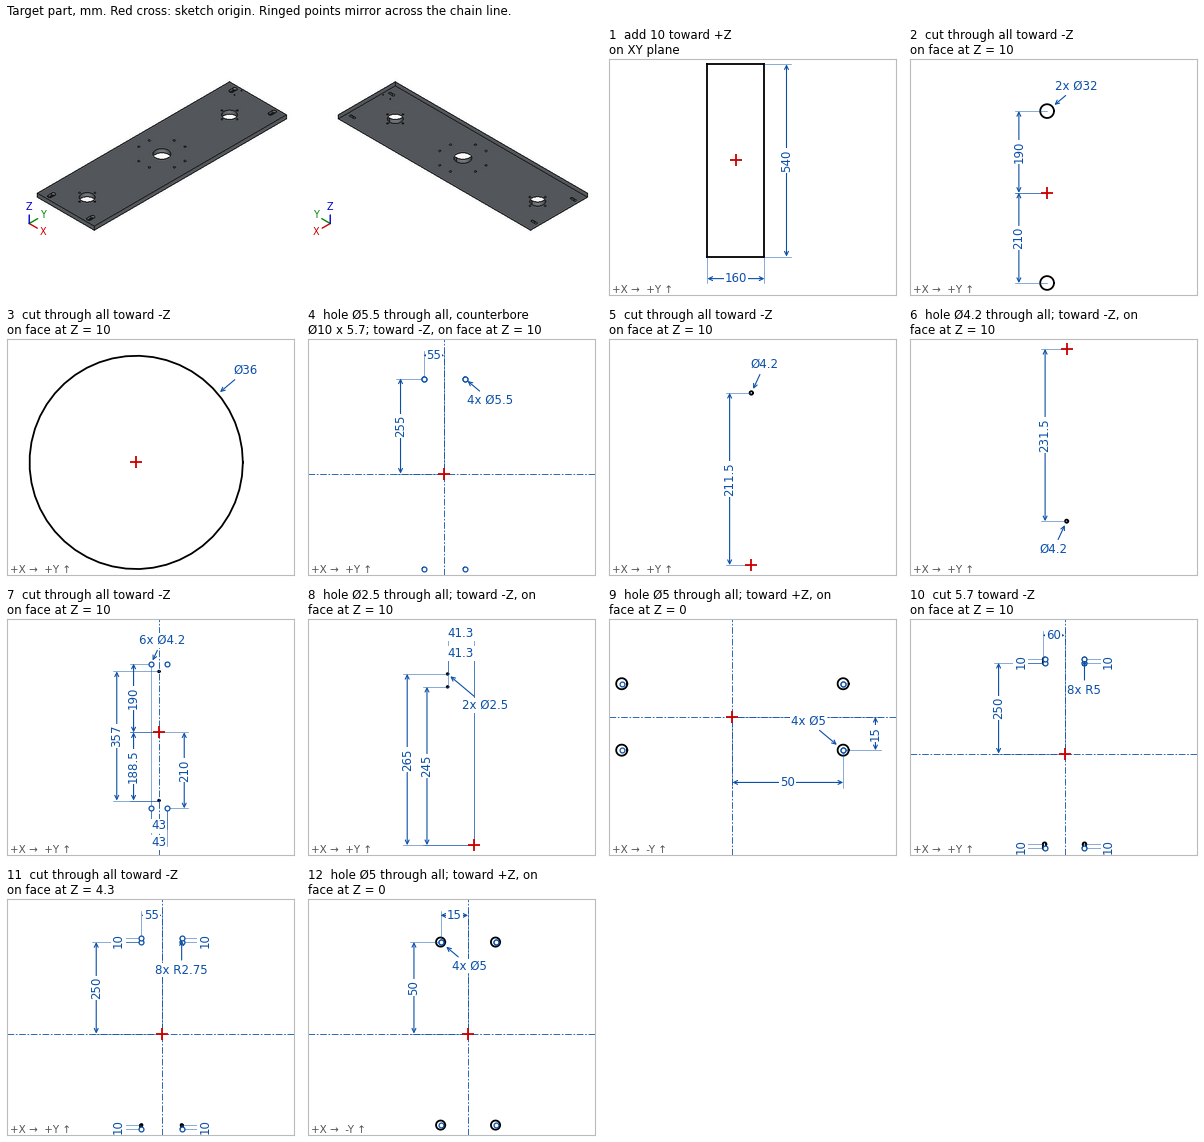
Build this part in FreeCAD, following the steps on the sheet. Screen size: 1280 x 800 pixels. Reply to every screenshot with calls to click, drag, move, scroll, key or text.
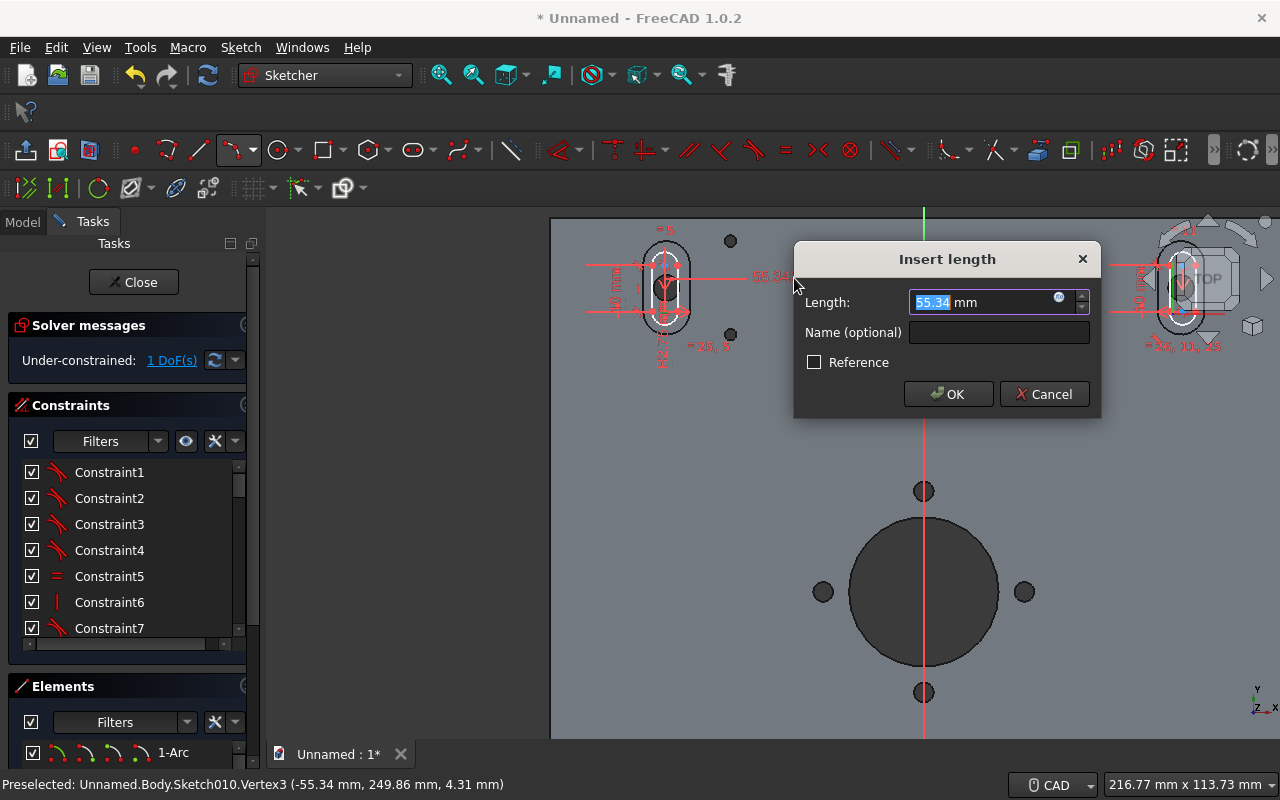
text(55)
key(Return)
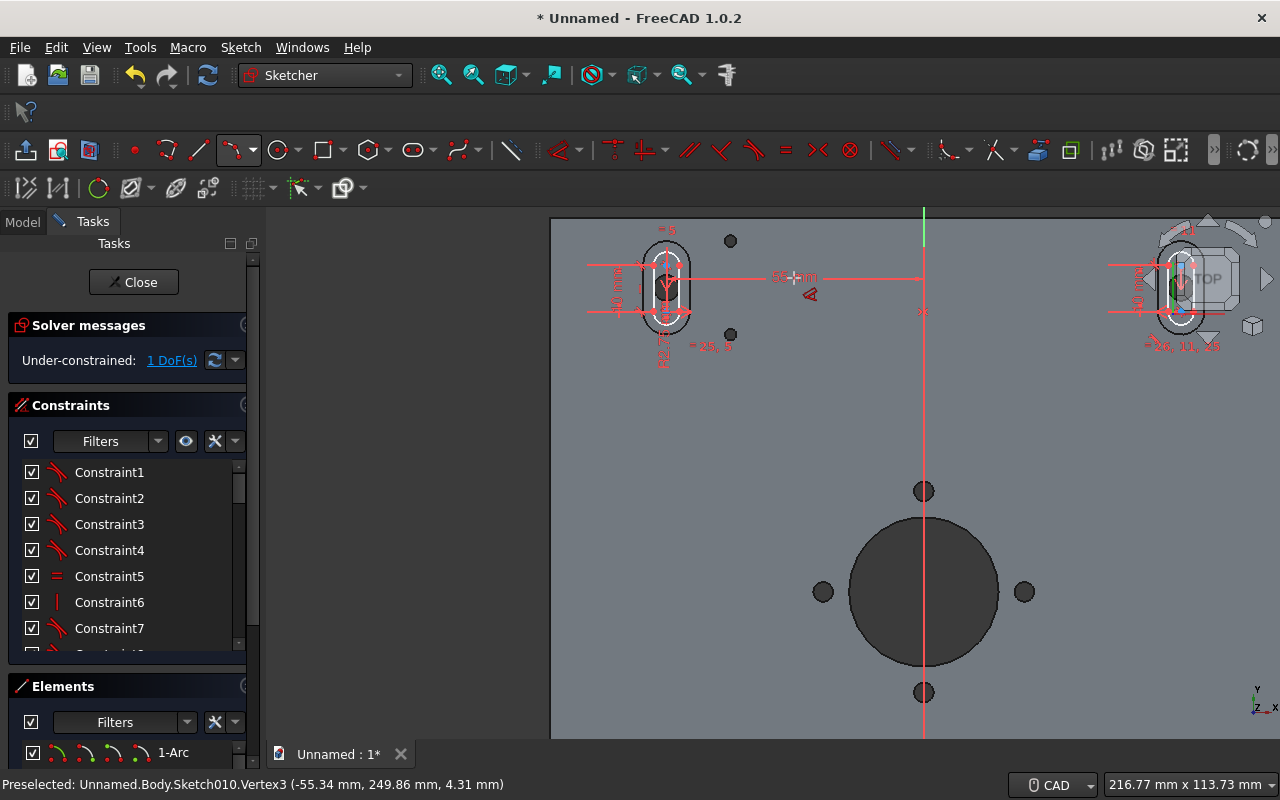
click(654, 312)
click(620, 511)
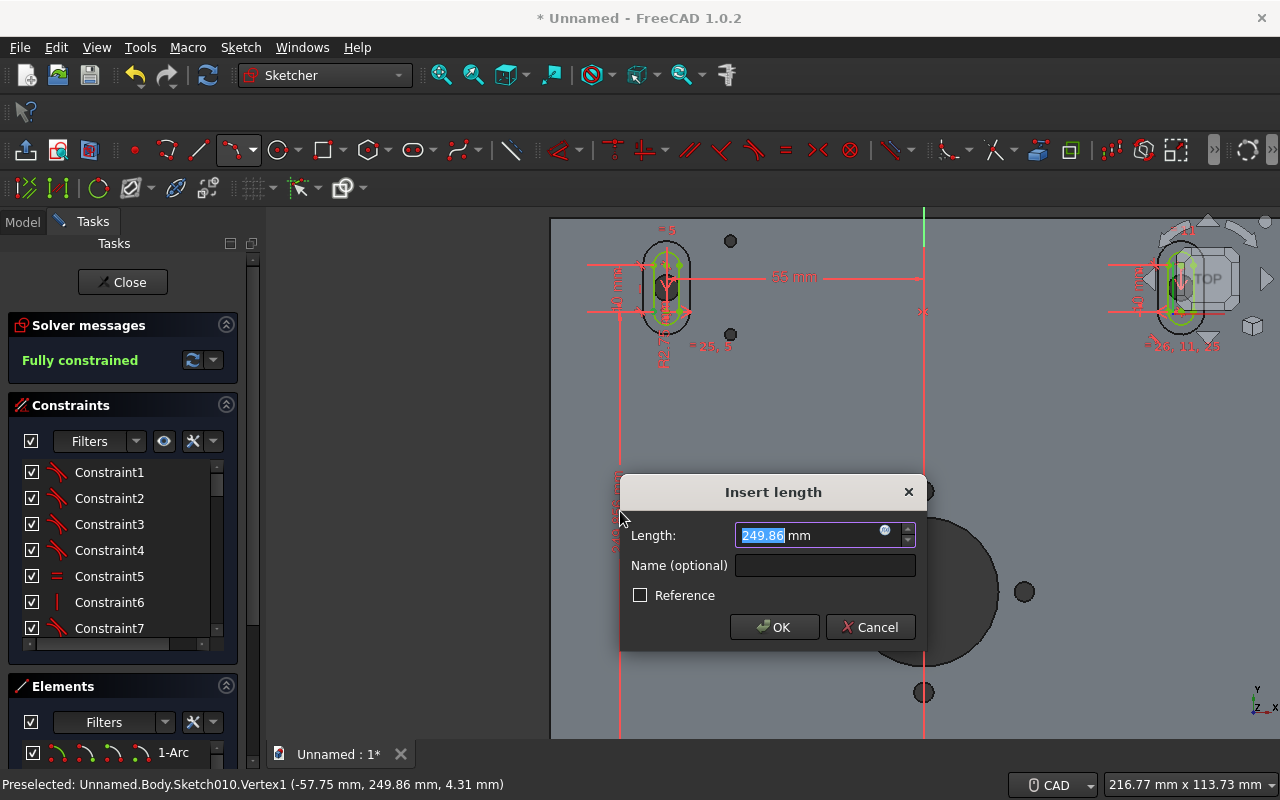
text(250)
key(Return)
key(Escape)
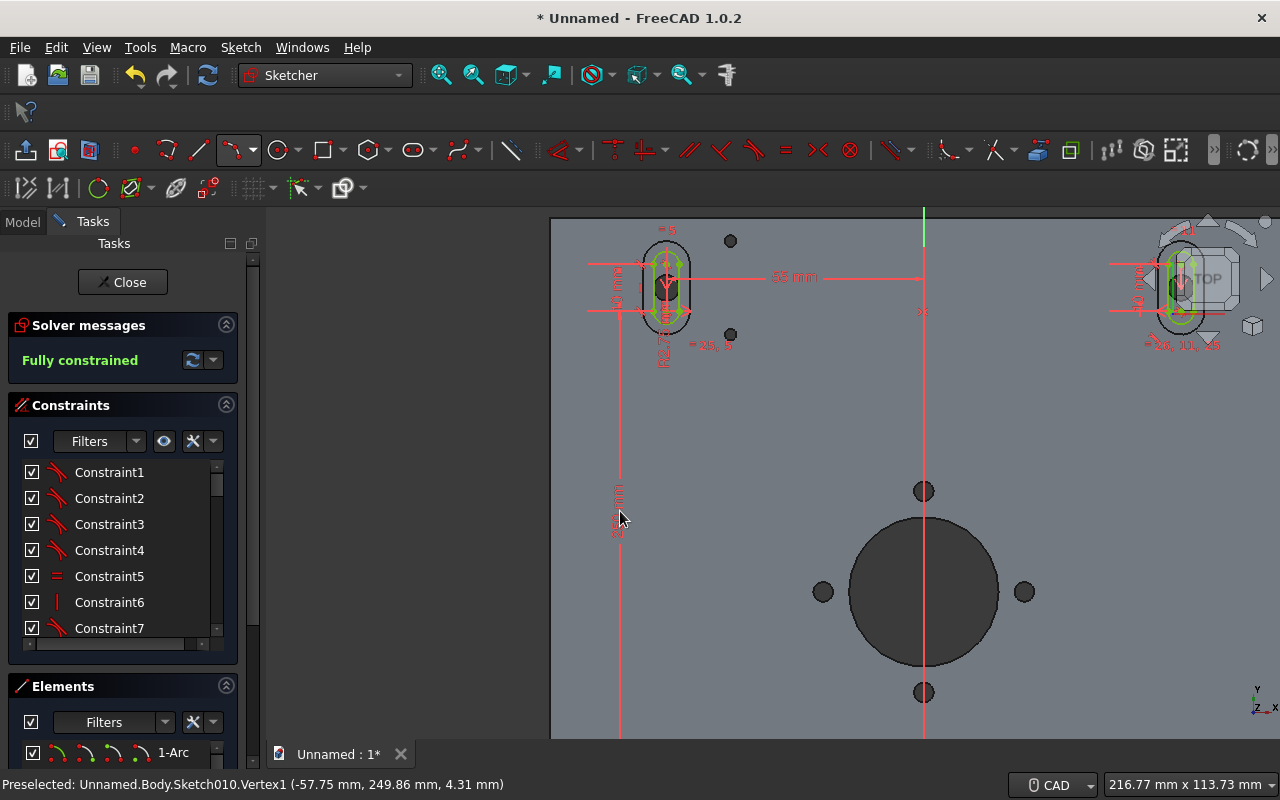
click(123, 282)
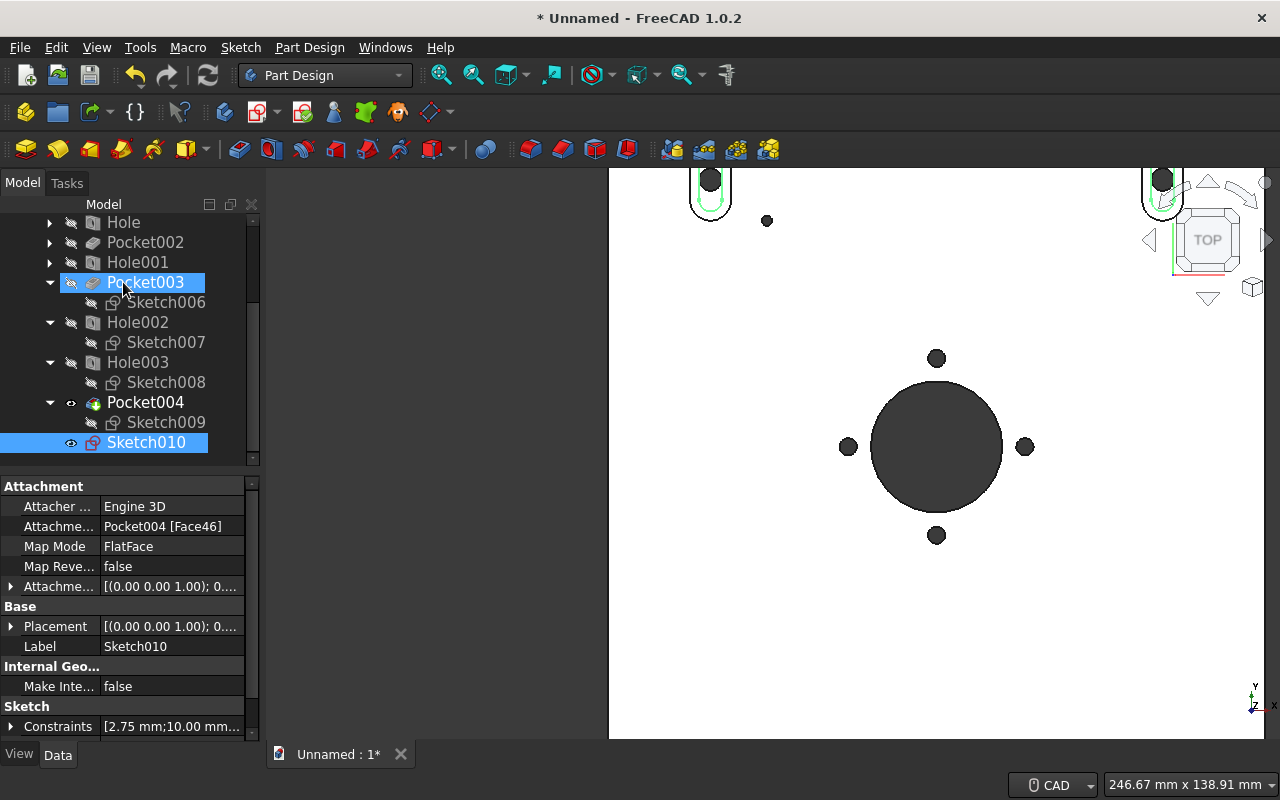
click(240, 150)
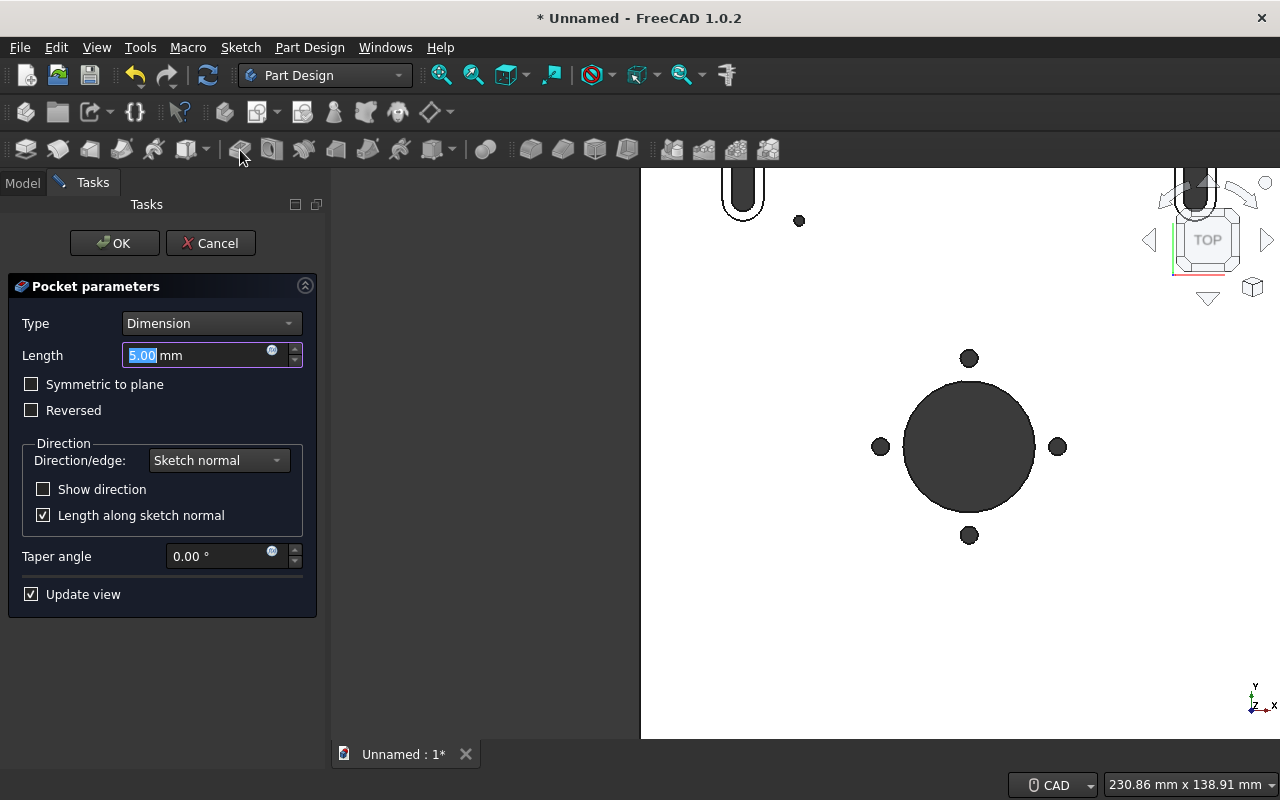
click(212, 324)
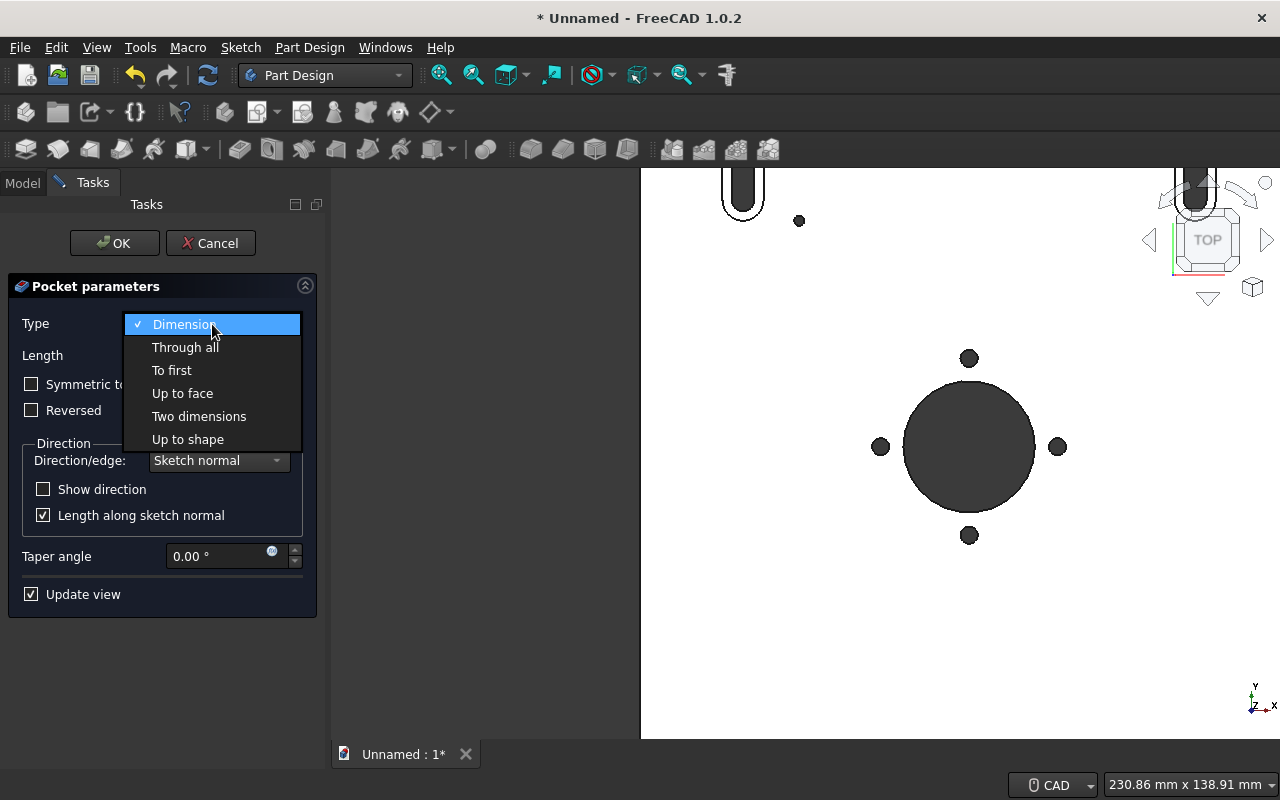
click(212, 348)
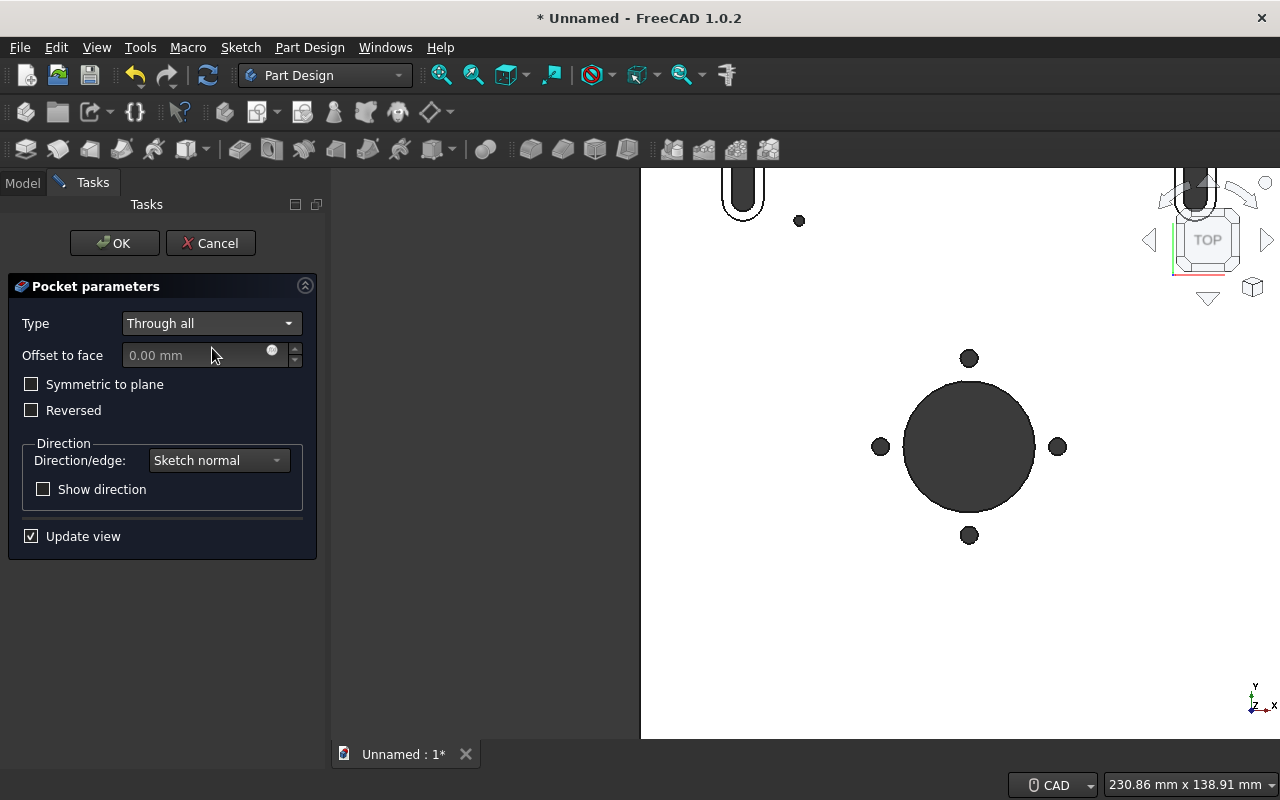
click(115, 243)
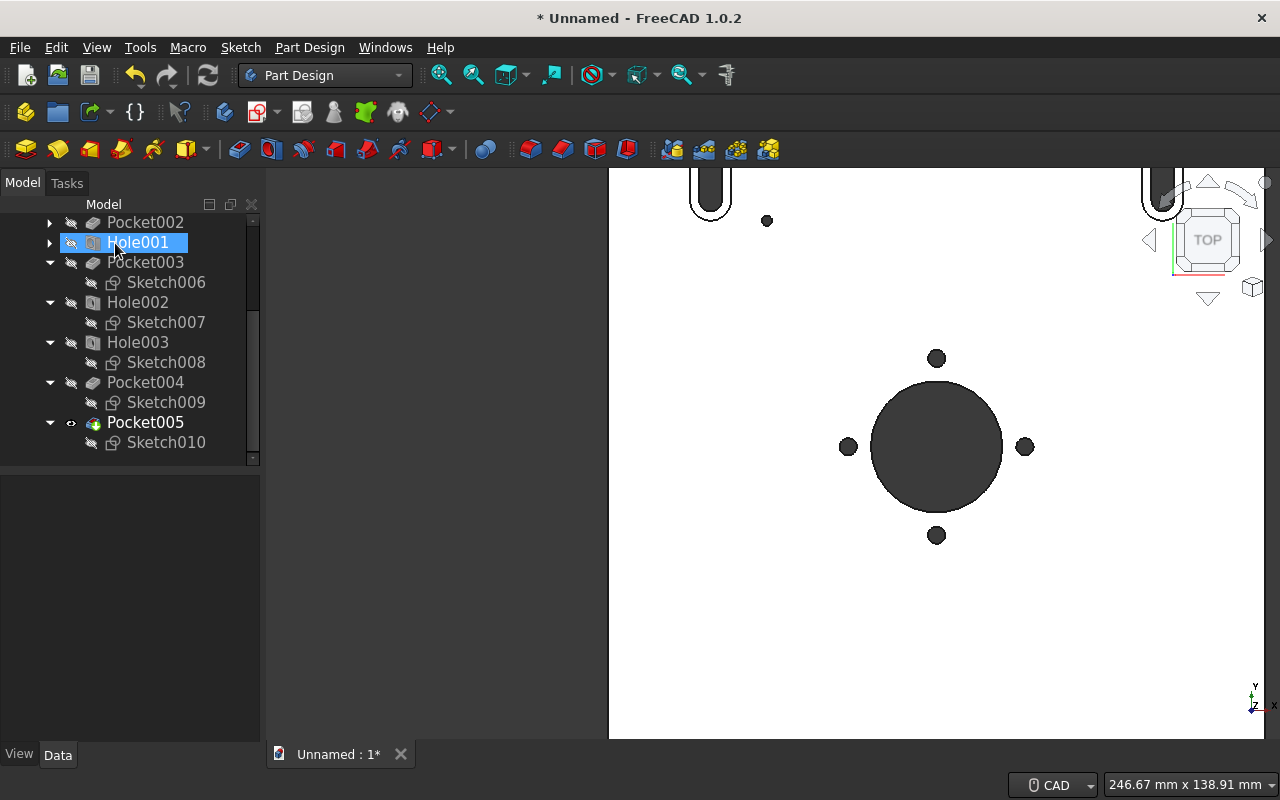
key(v)
key(f)